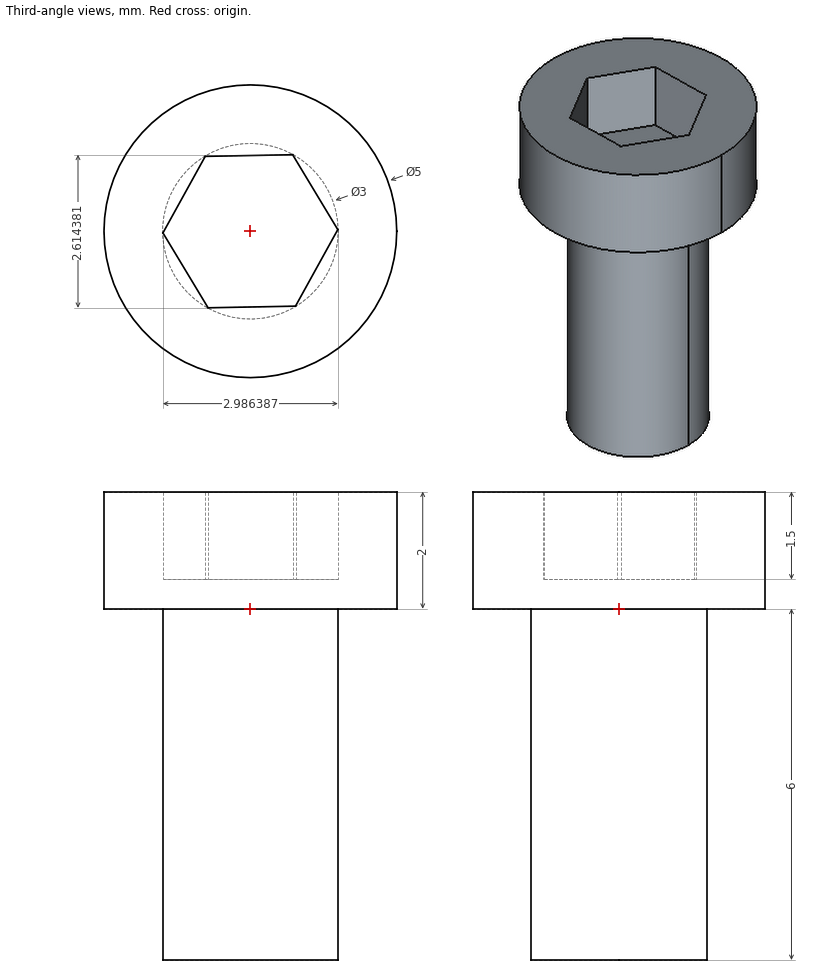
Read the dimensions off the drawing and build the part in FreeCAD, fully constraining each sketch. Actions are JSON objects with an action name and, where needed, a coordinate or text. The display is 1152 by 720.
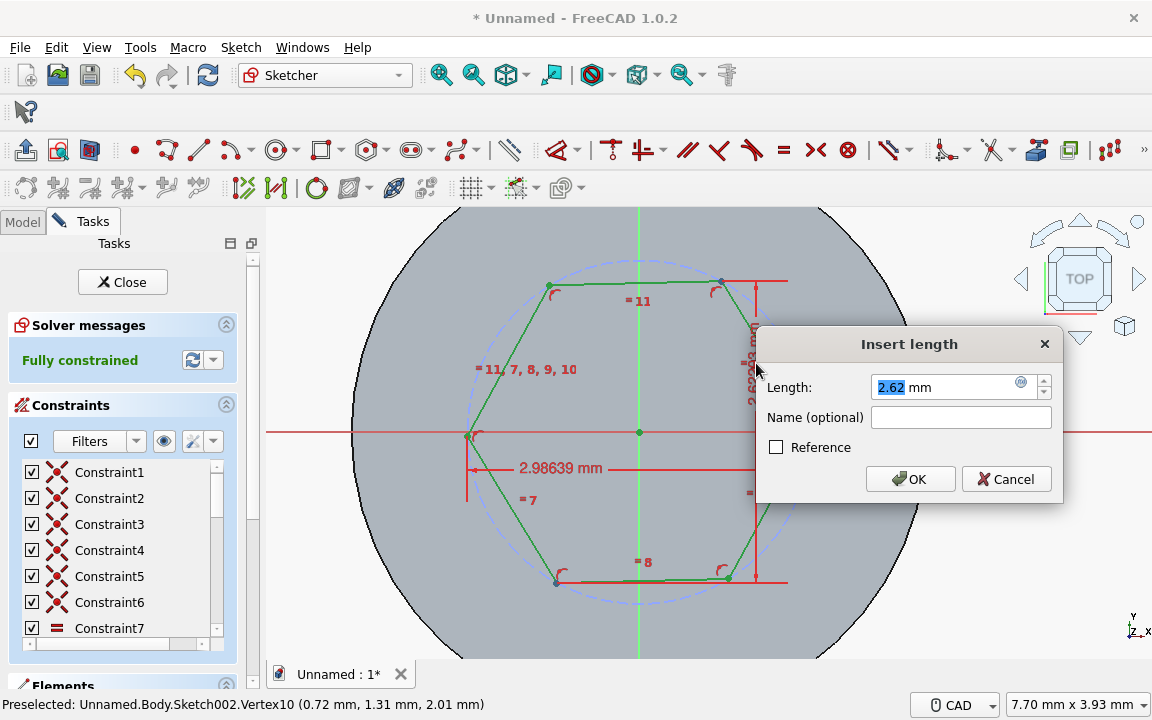
{"action": "type", "text": "2.614381"}
{"action": "key", "text": "Return"}
{"action": "key", "text": "Escape"}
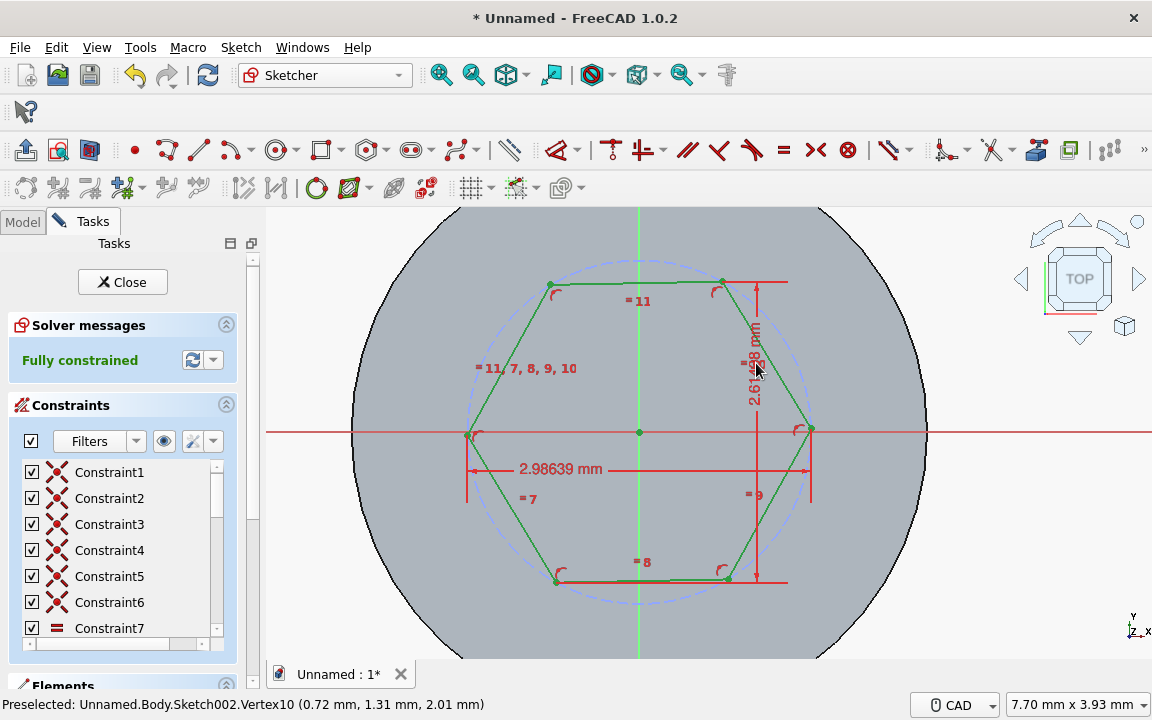
{"action": "left_click", "coordinate": [123, 282]}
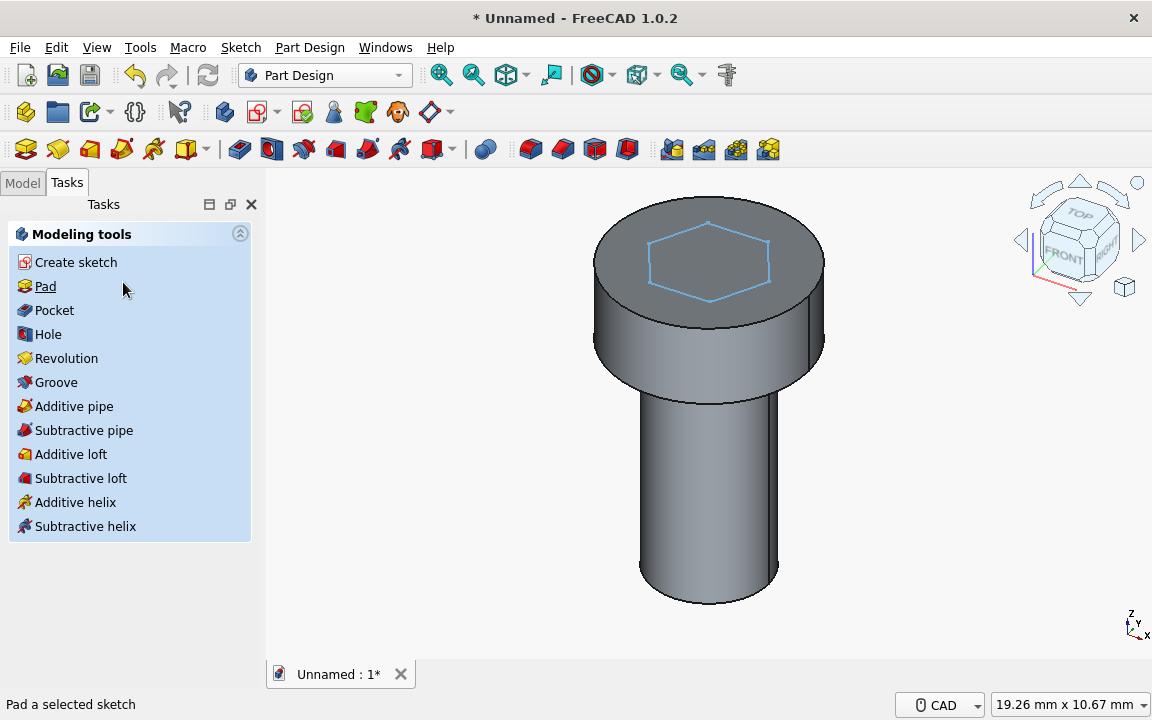
{"action": "left_click", "coordinate": [240, 150]}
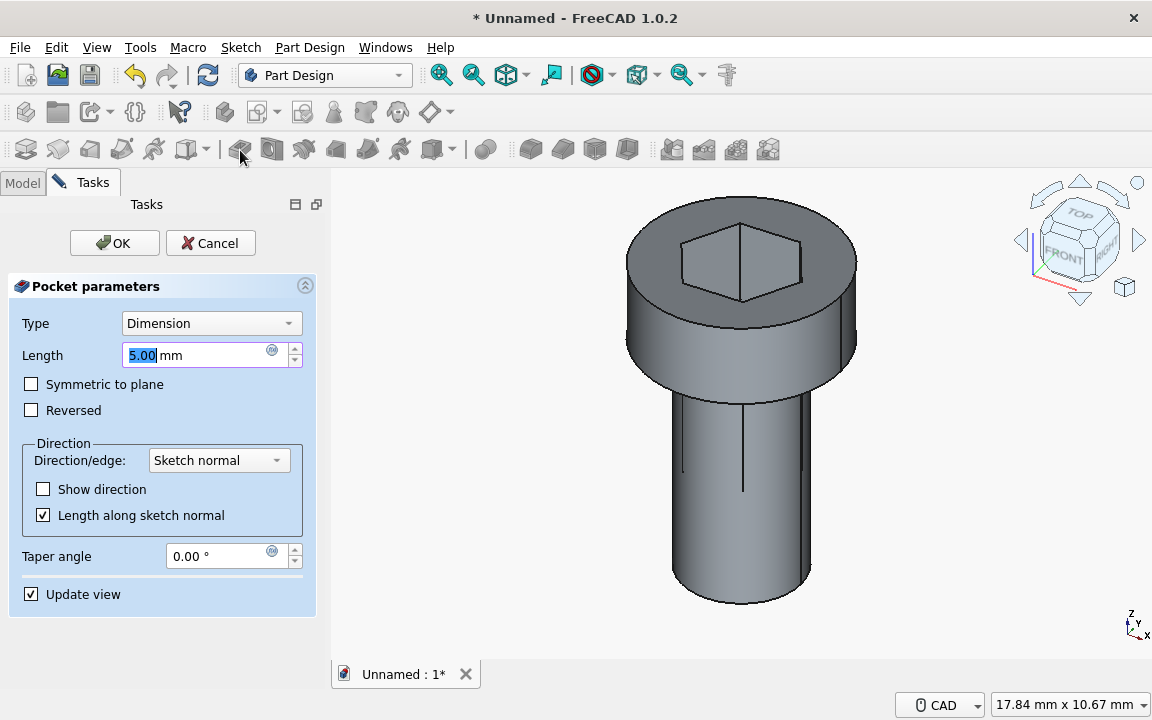
{"action": "type", "text": "1.5"}
{"action": "key", "text": "Tab"}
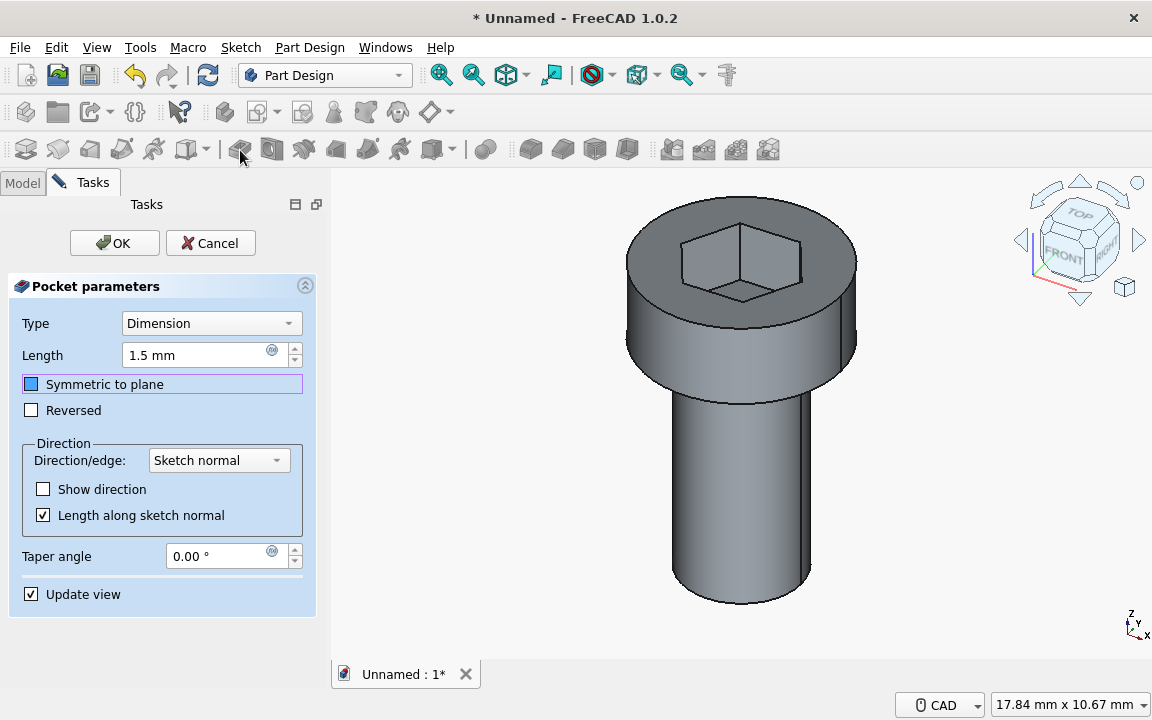
{"action": "left_click", "coordinate": [115, 243]}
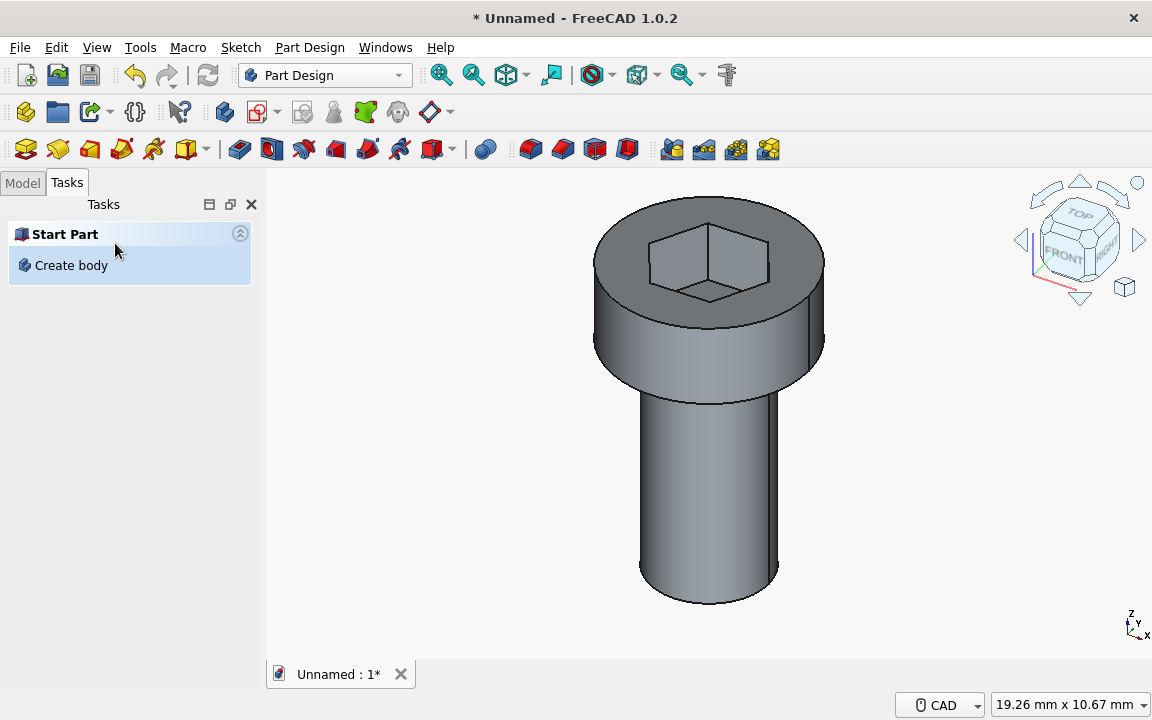
{"action": "key", "text": "0"}